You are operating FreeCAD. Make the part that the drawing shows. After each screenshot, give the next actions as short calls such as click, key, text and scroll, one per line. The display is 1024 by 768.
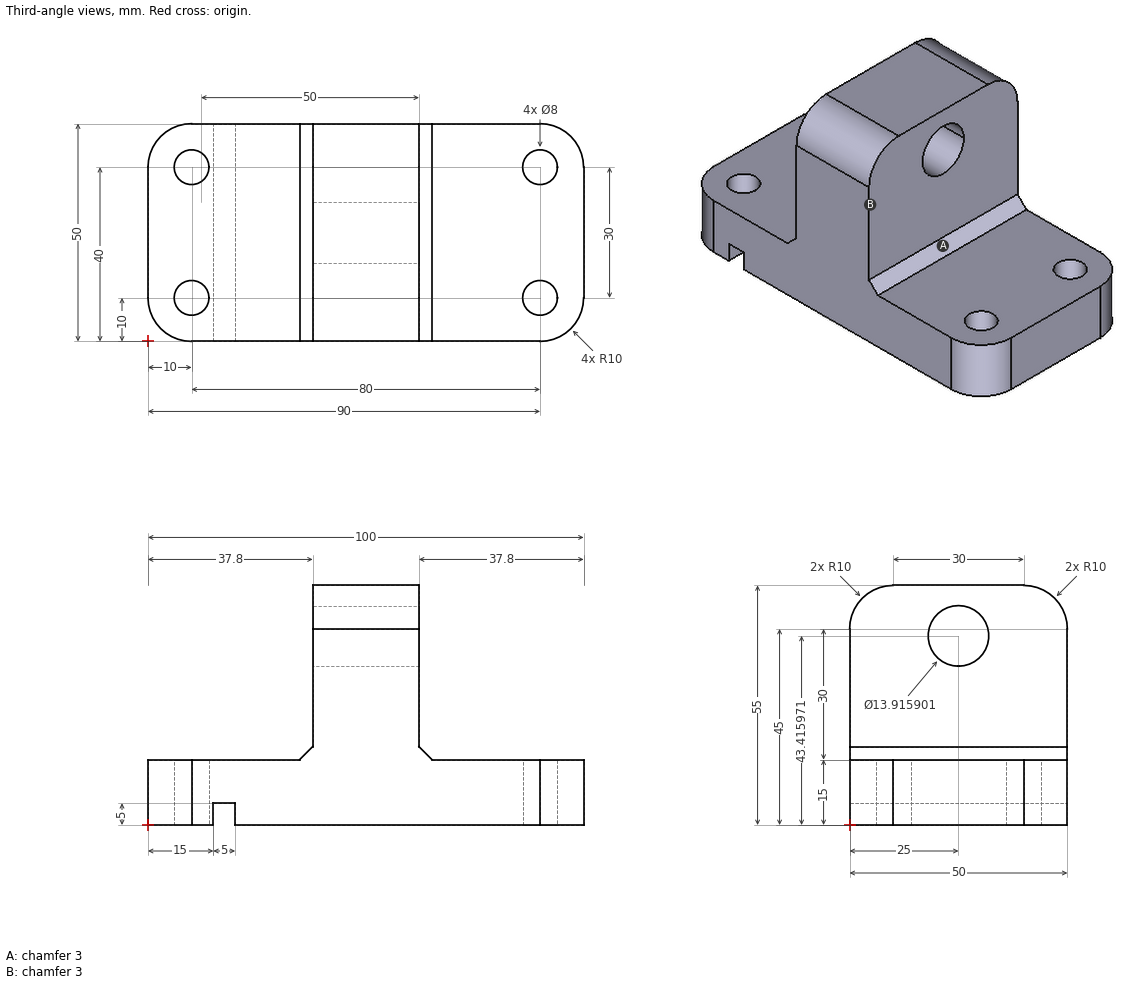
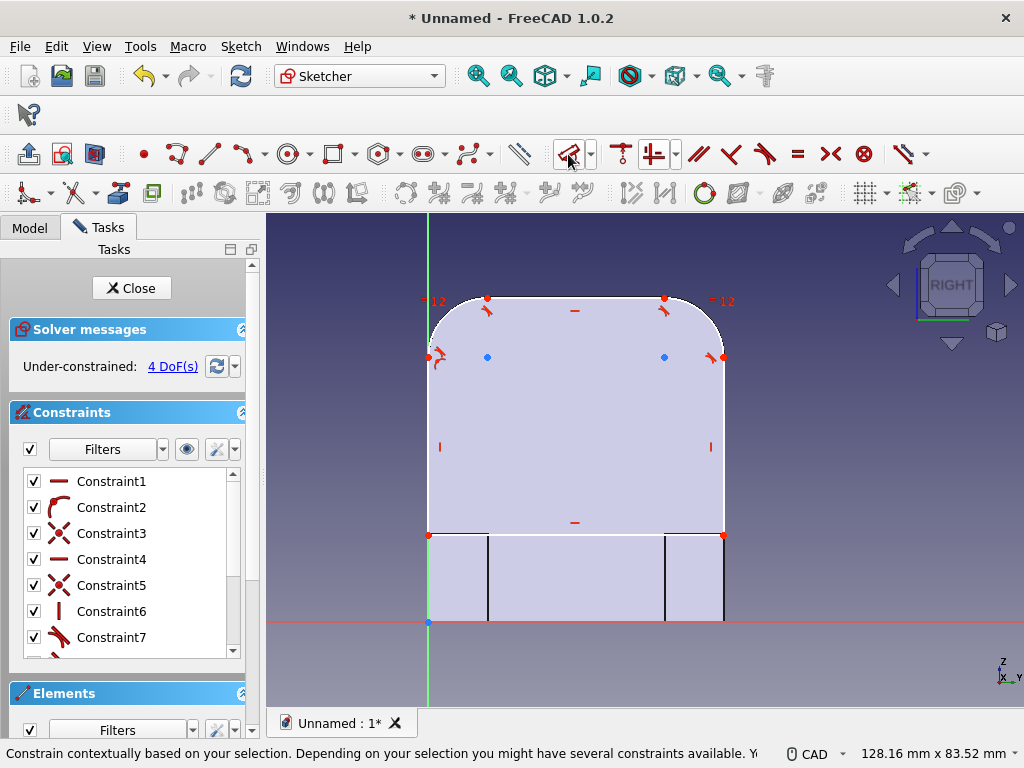
click(461, 305)
click(447, 276)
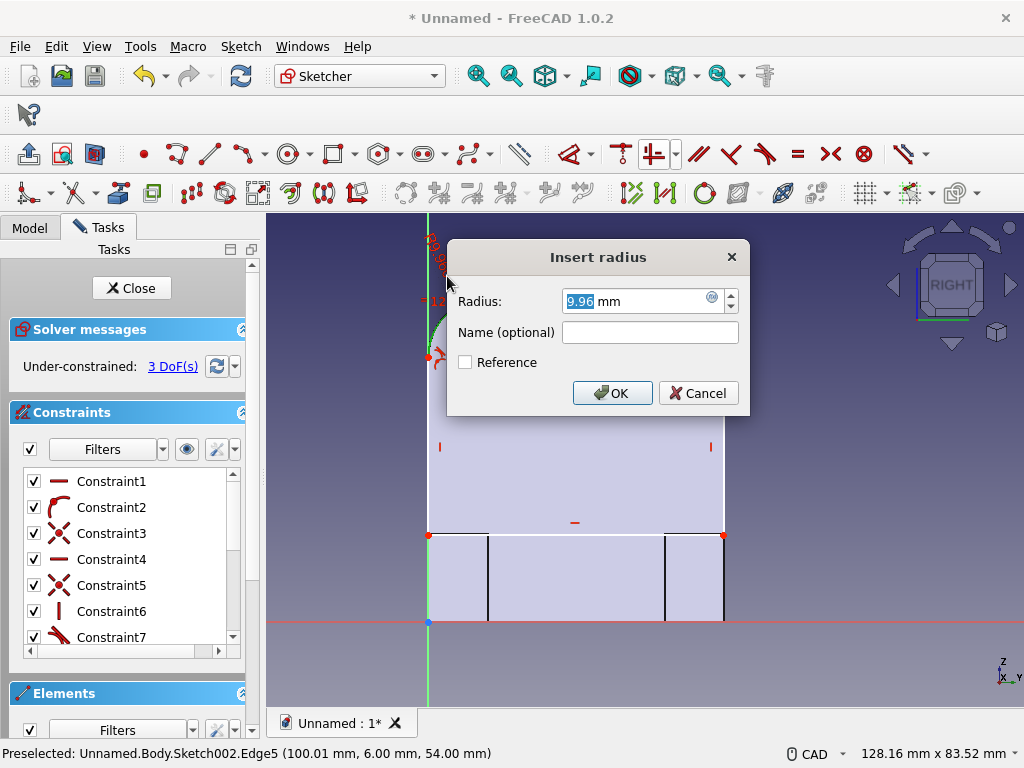
text(10)
key(Return)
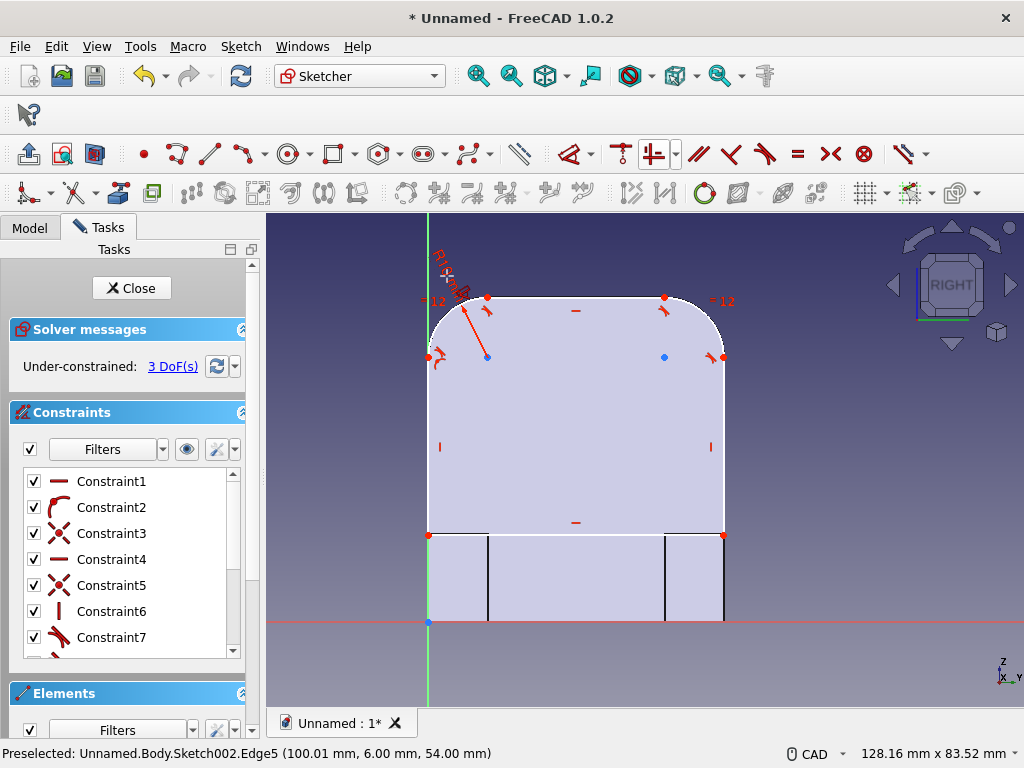
click(612, 298)
click(576, 264)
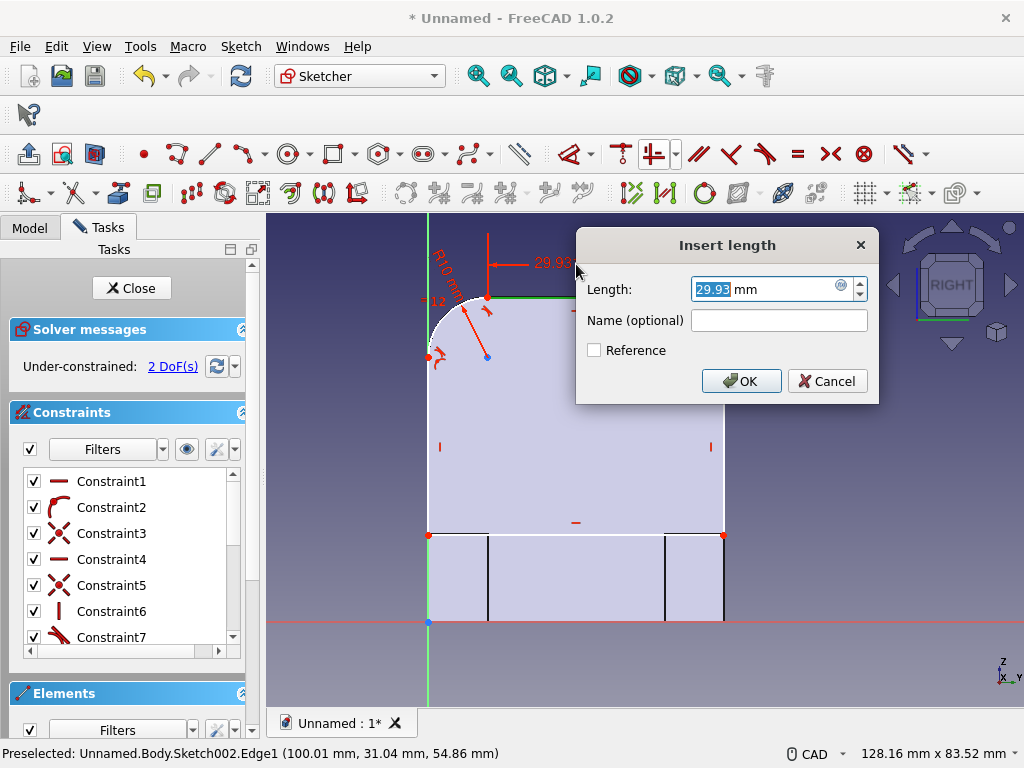
text(30)
key(Return)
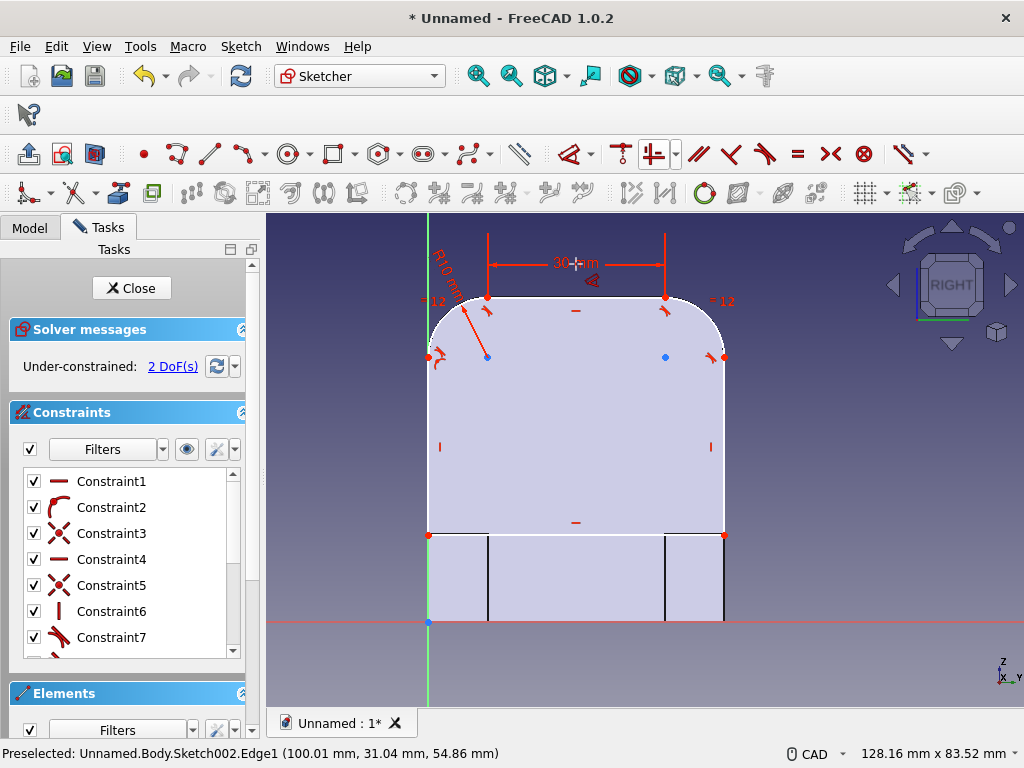
click(428, 410)
click(394, 446)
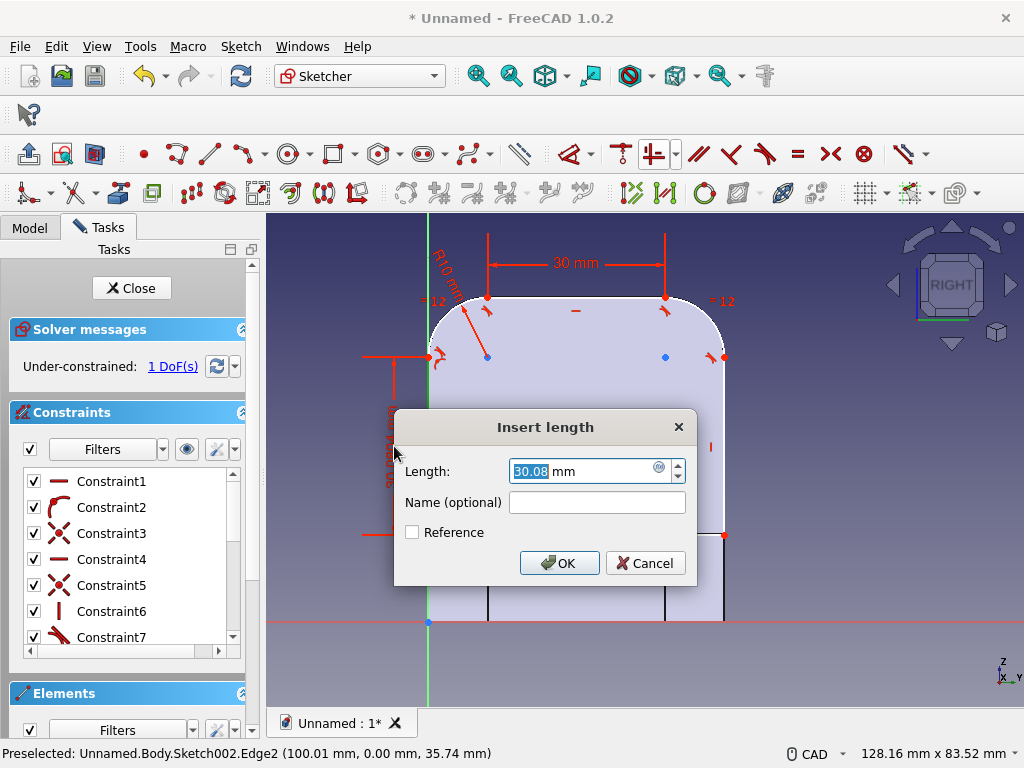
text(30)
key(Return)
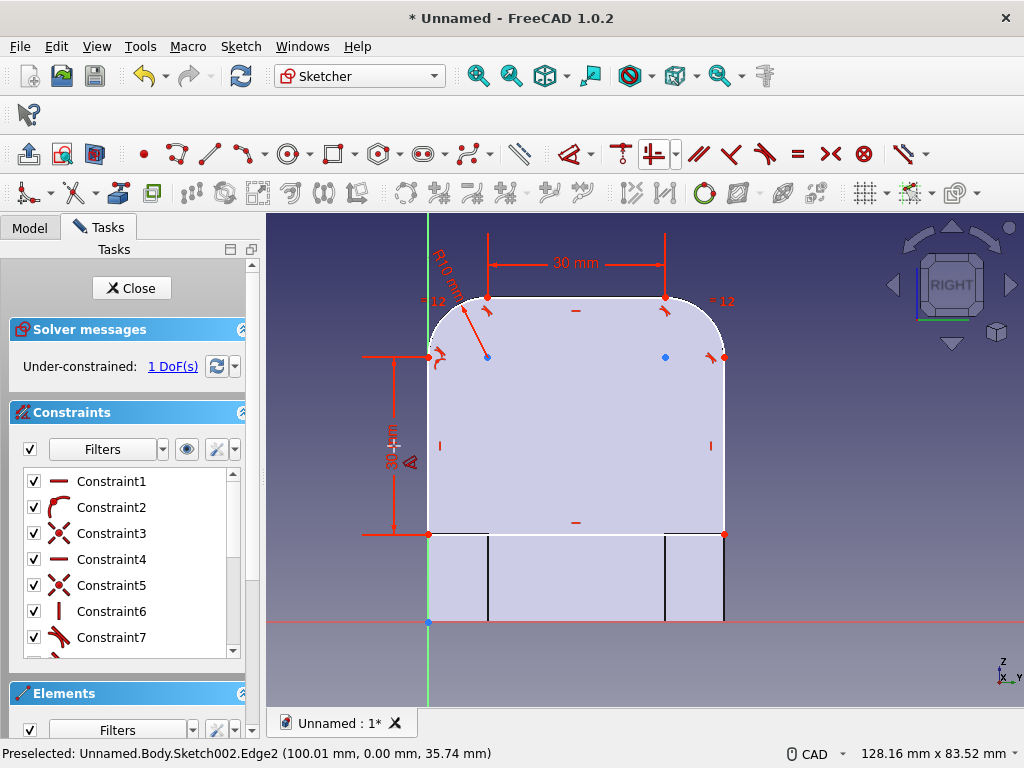
click(665, 298)
click(394, 386)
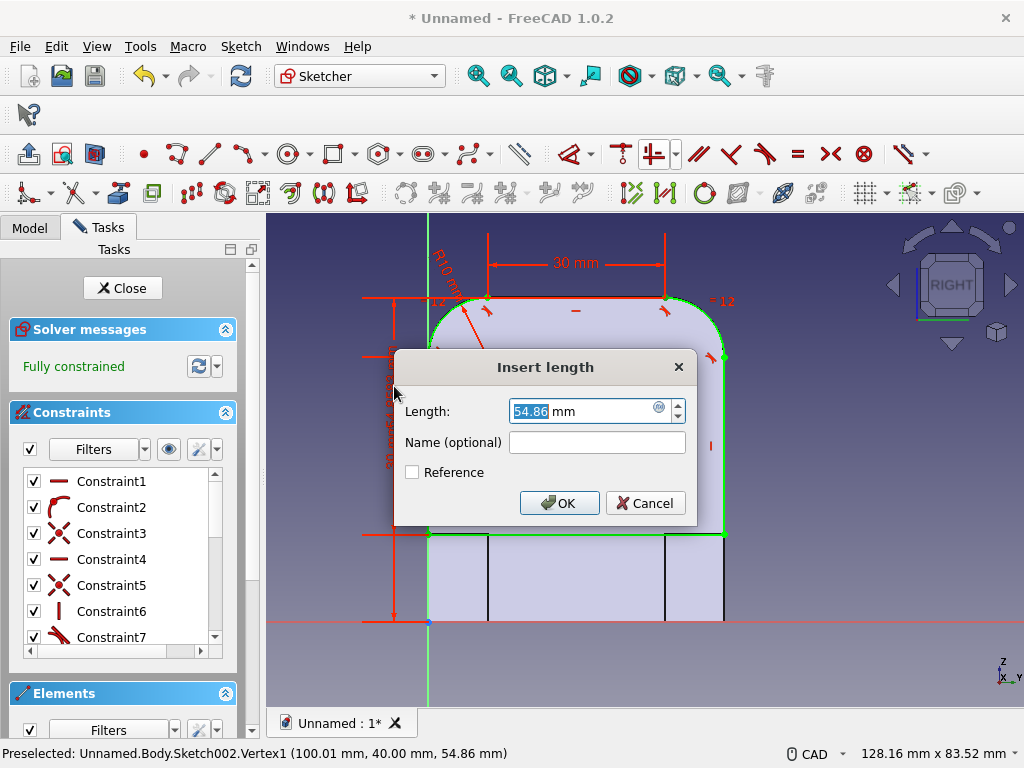
text(55)
key(Return)
key(Escape)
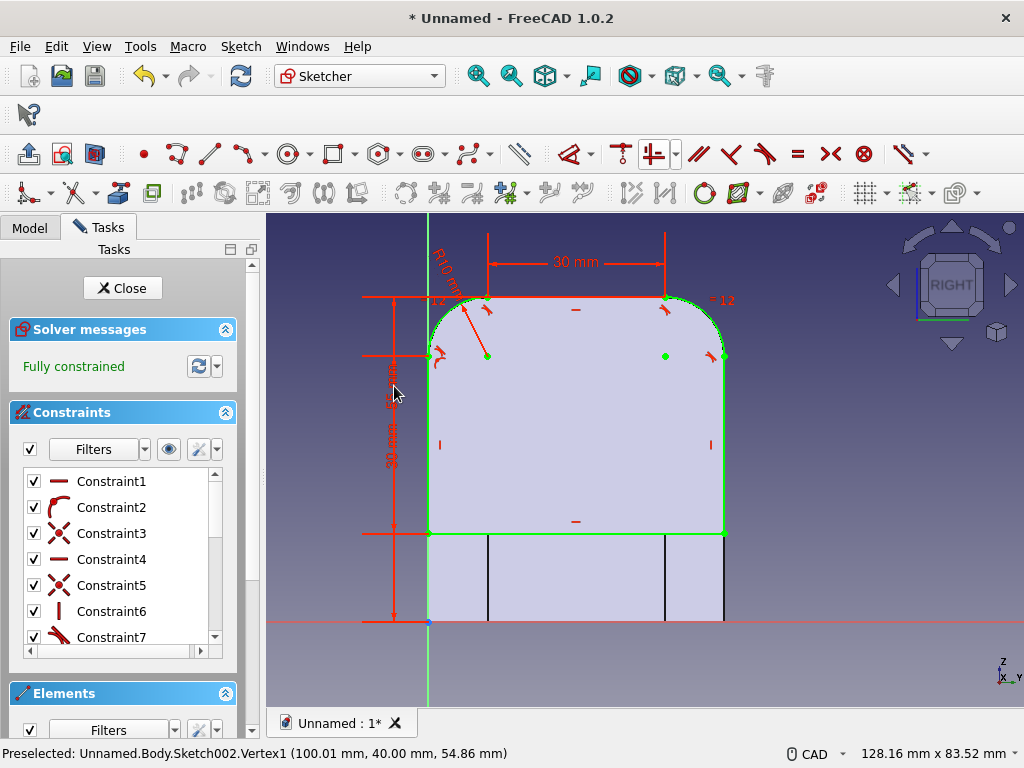
click(123, 288)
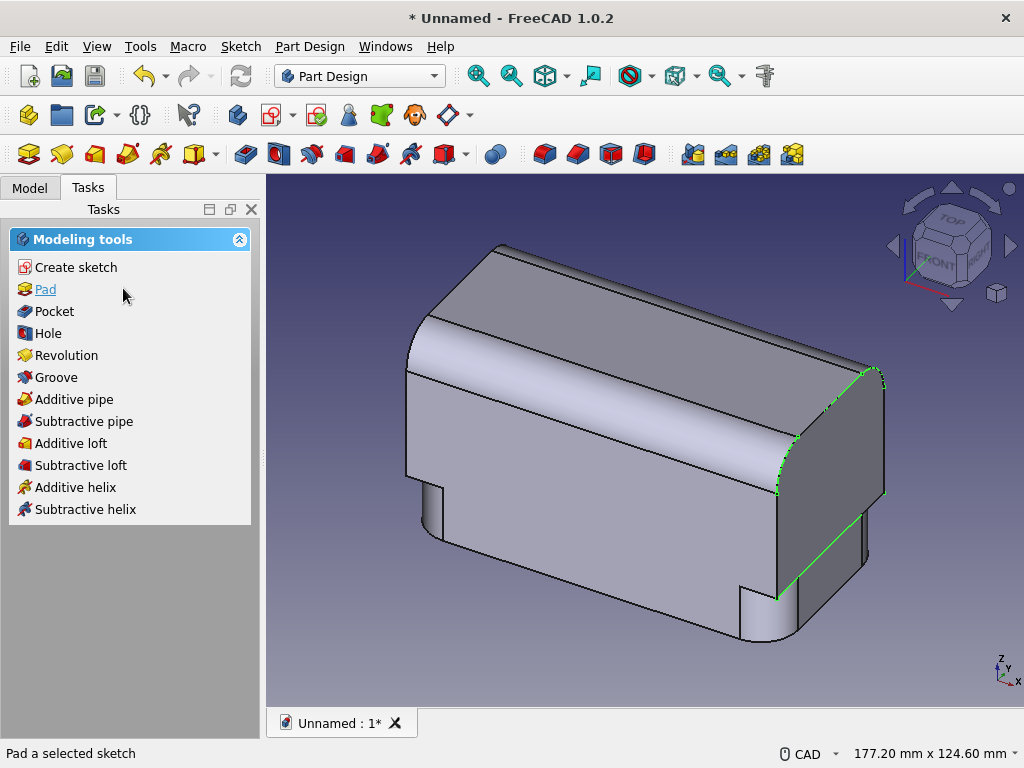
click(246, 154)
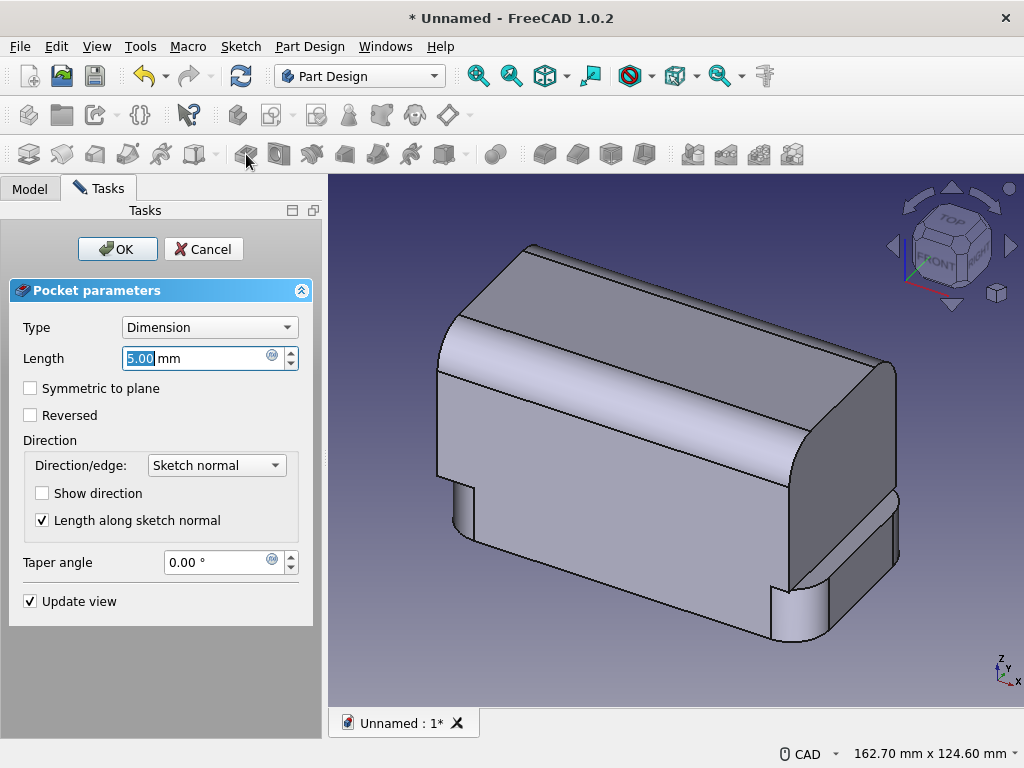
text(37.8)
key(Tab)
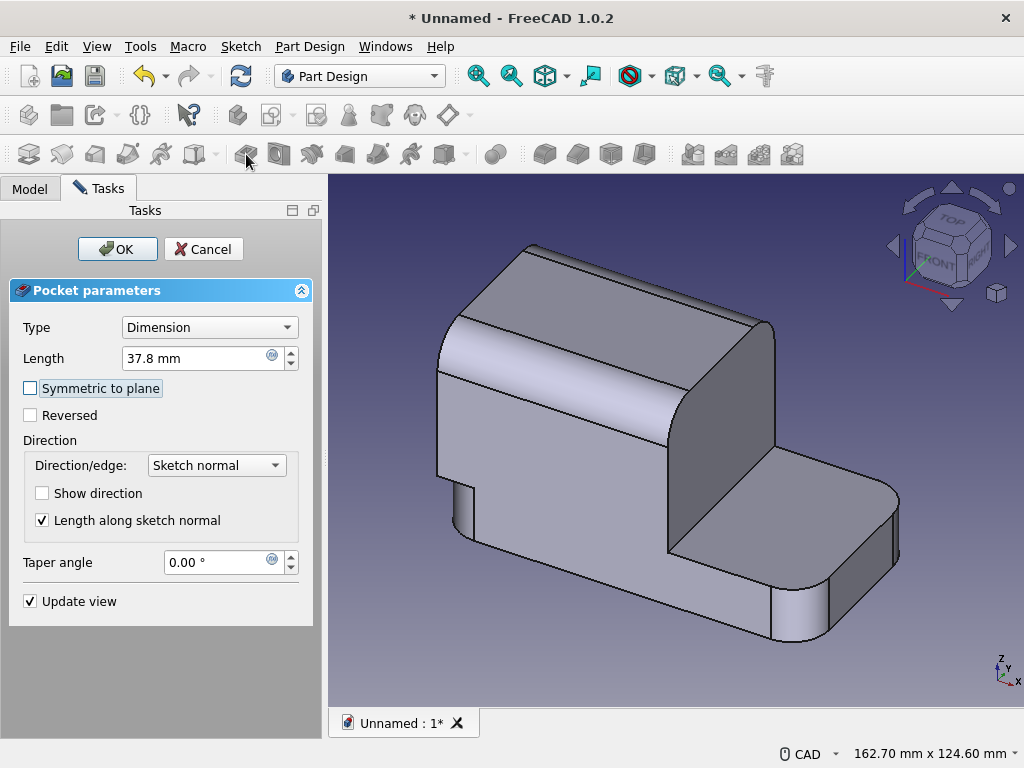
click(118, 249)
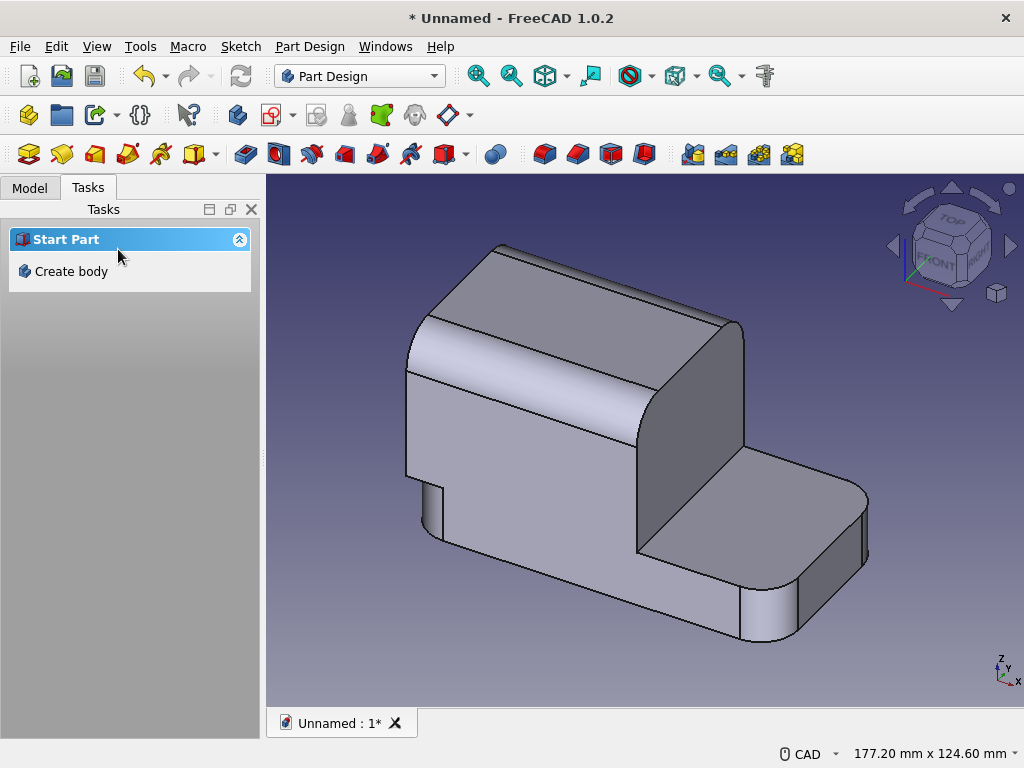
click(30, 188)